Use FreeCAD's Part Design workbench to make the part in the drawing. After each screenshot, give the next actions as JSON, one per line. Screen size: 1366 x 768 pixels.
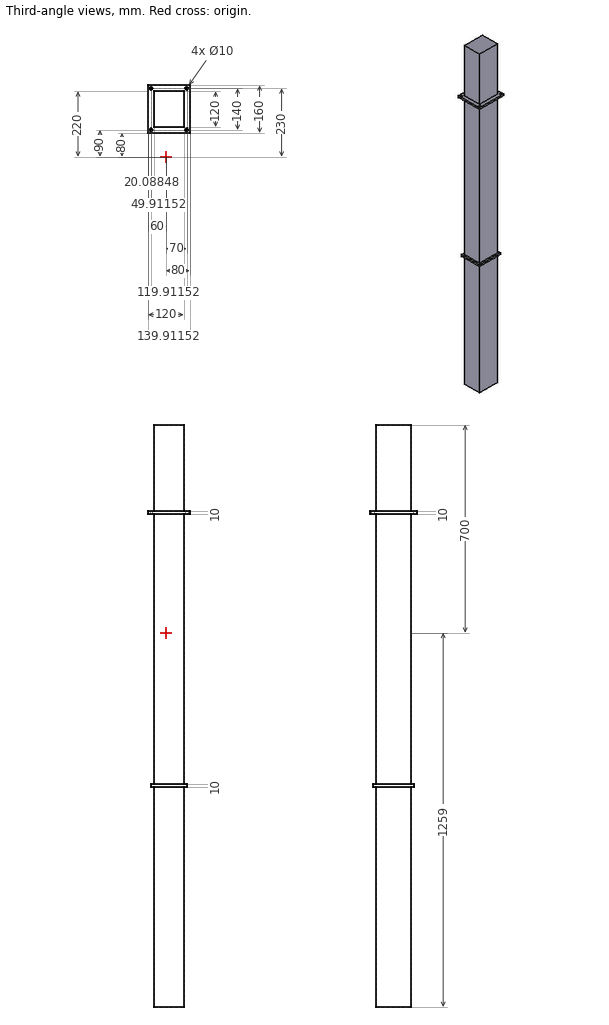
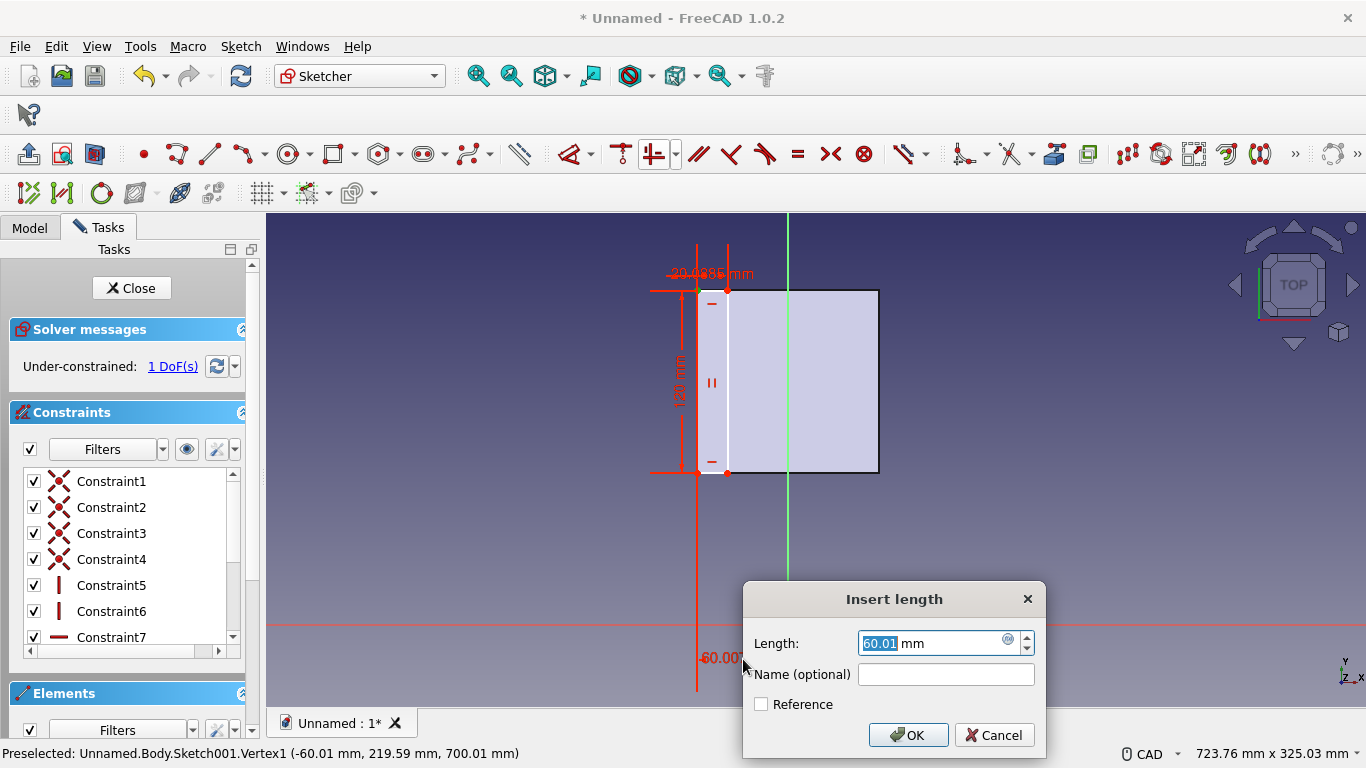
{"action": "type", "text": "60"}
{"action": "key", "text": "Return"}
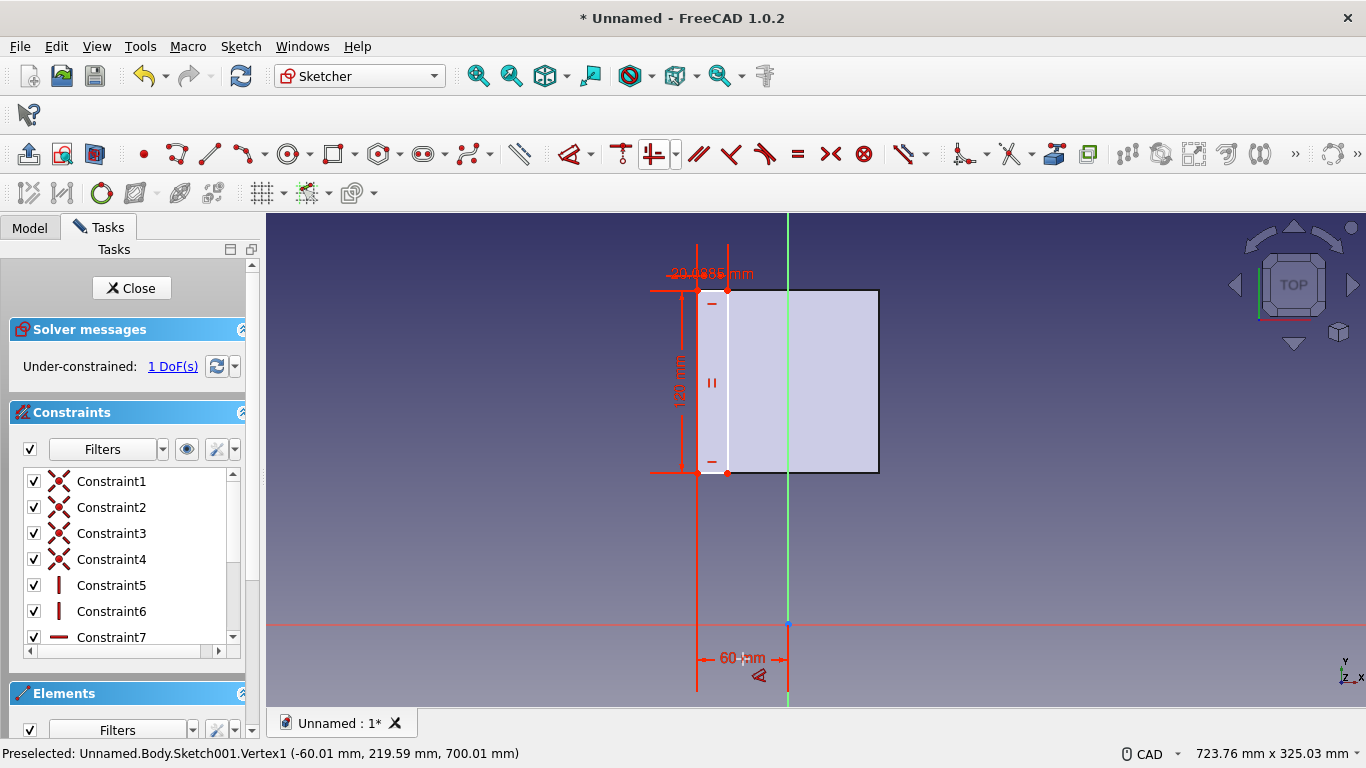
{"action": "left_click", "coordinate": [697, 291]}
{"action": "left_click", "coordinate": [822, 458]}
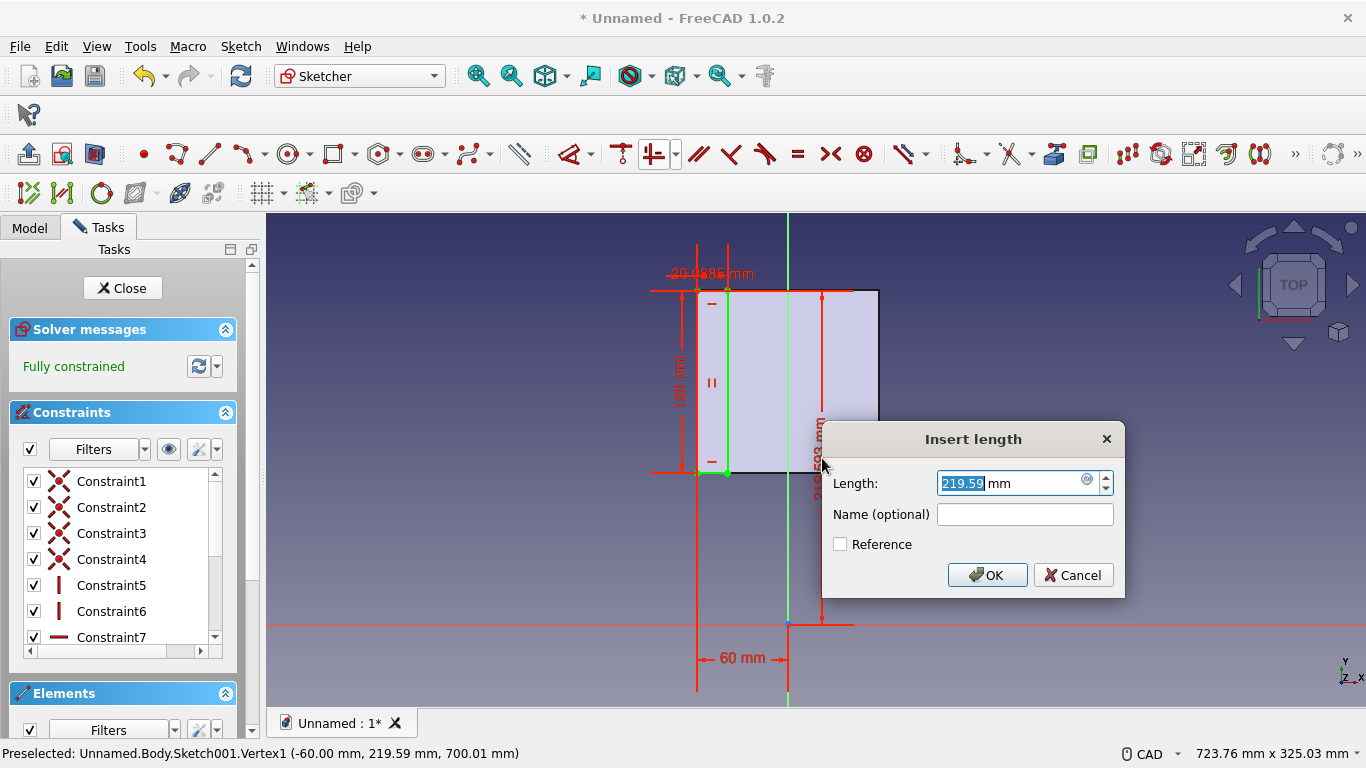
{"action": "type", "text": "220"}
{"action": "key", "text": "Return"}
{"action": "key", "text": "Escape"}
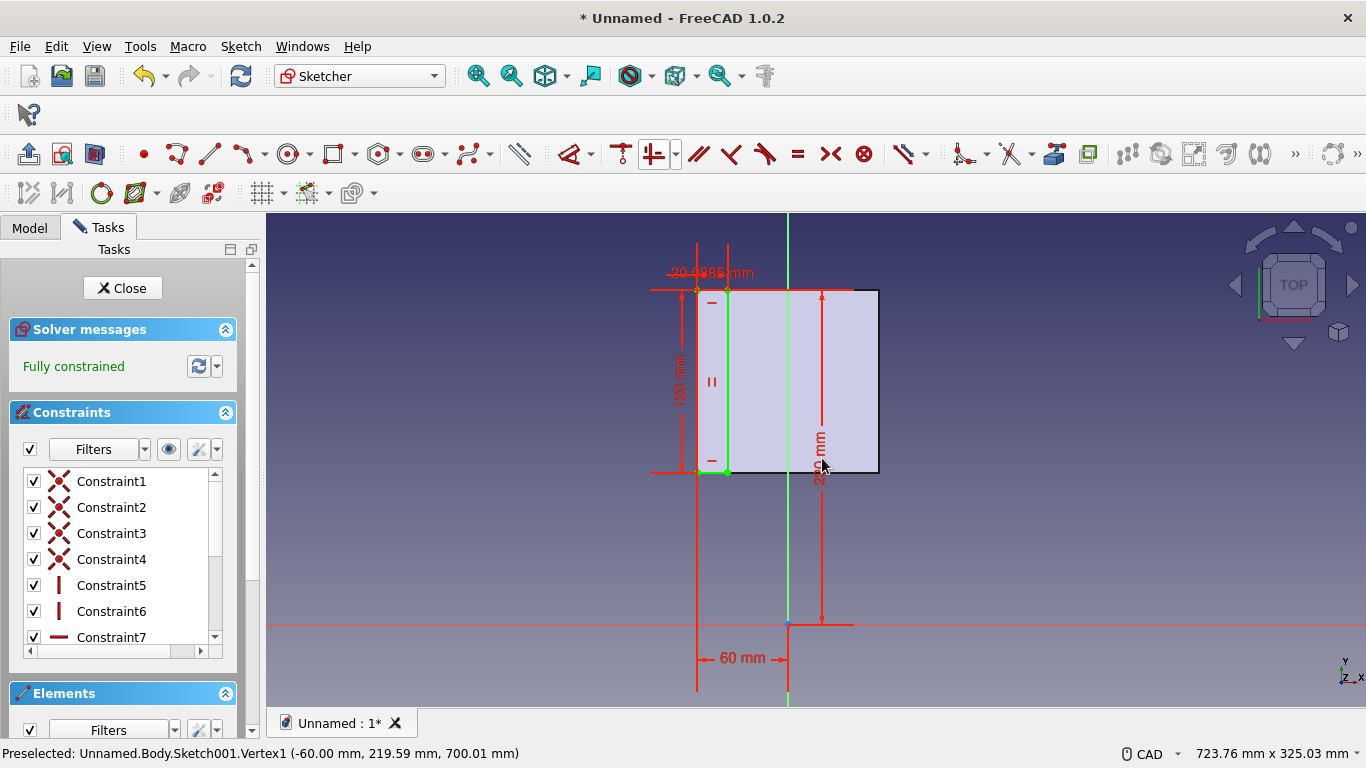
{"action": "left_click", "coordinate": [123, 288]}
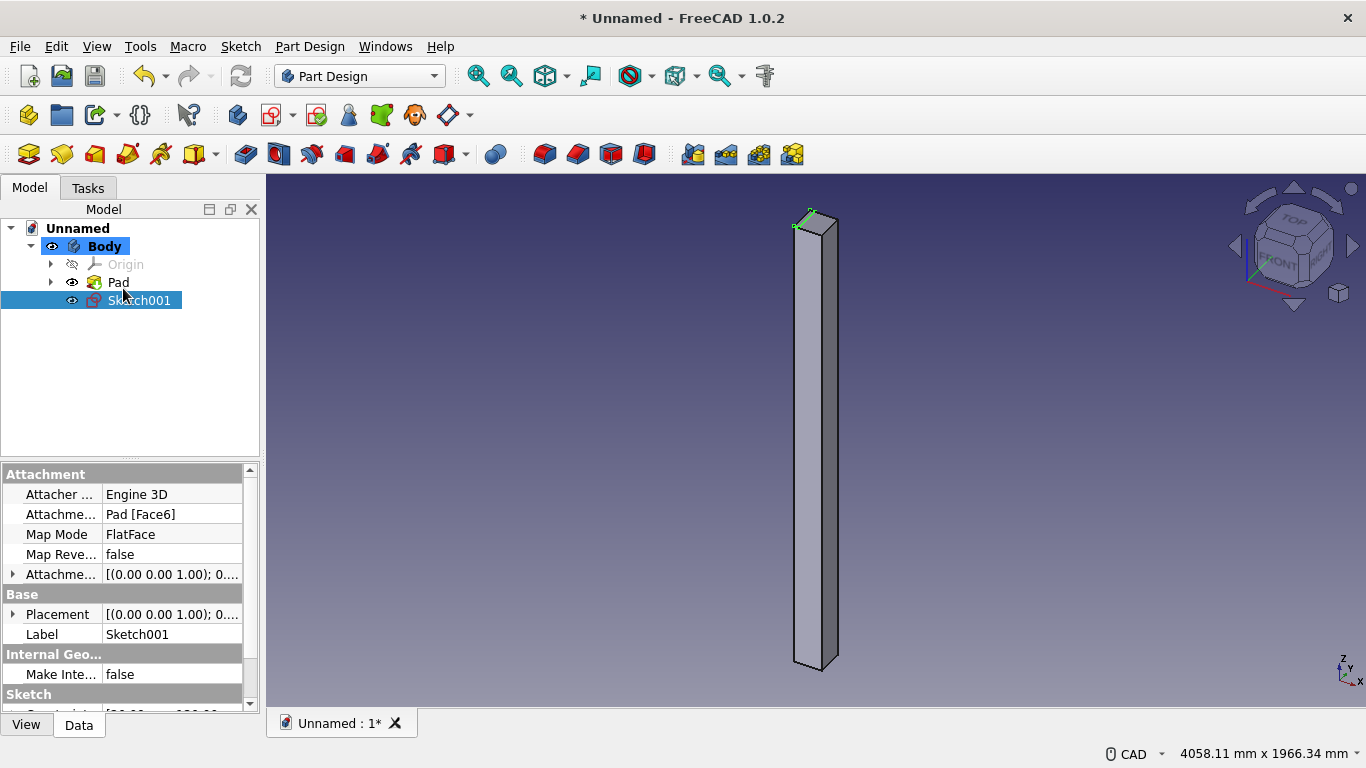
{"action": "left_click", "coordinate": [246, 154]}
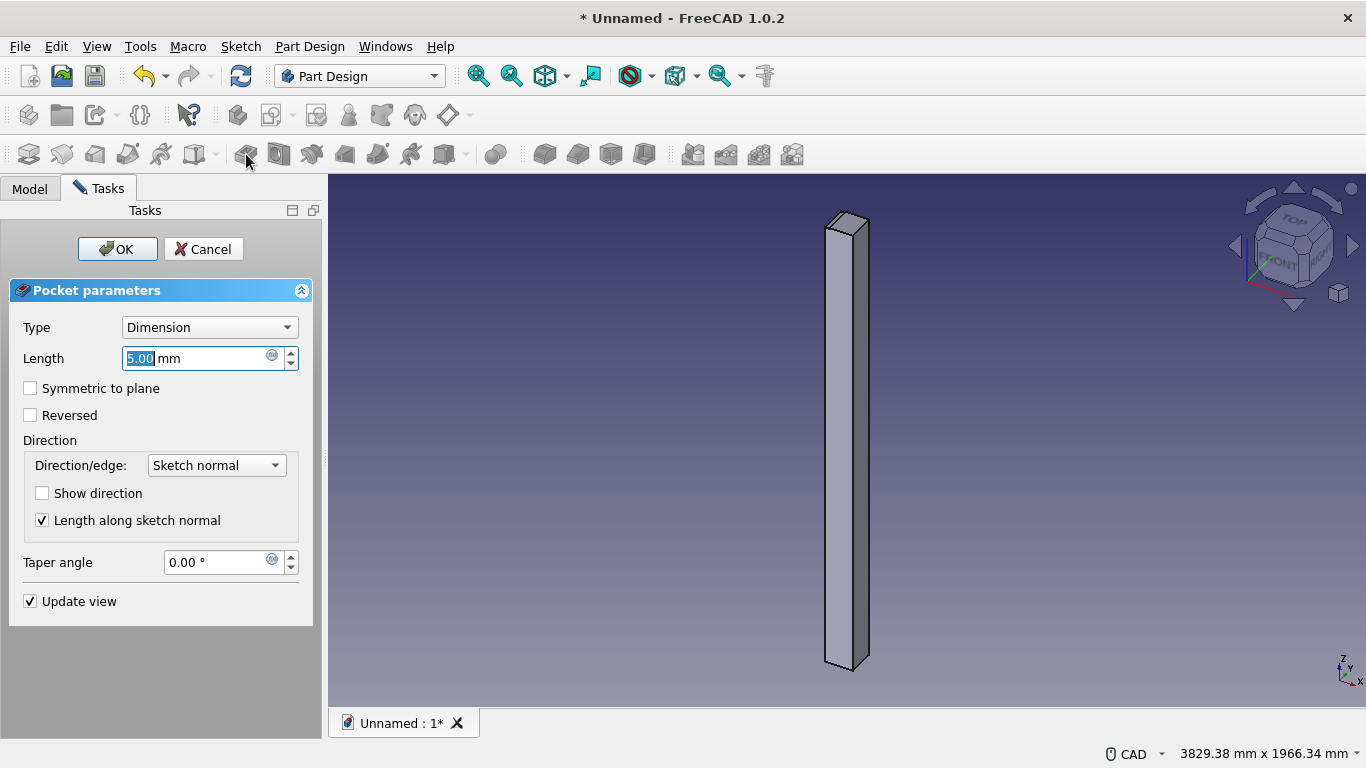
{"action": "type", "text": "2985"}
{"action": "key", "text": "Tab"}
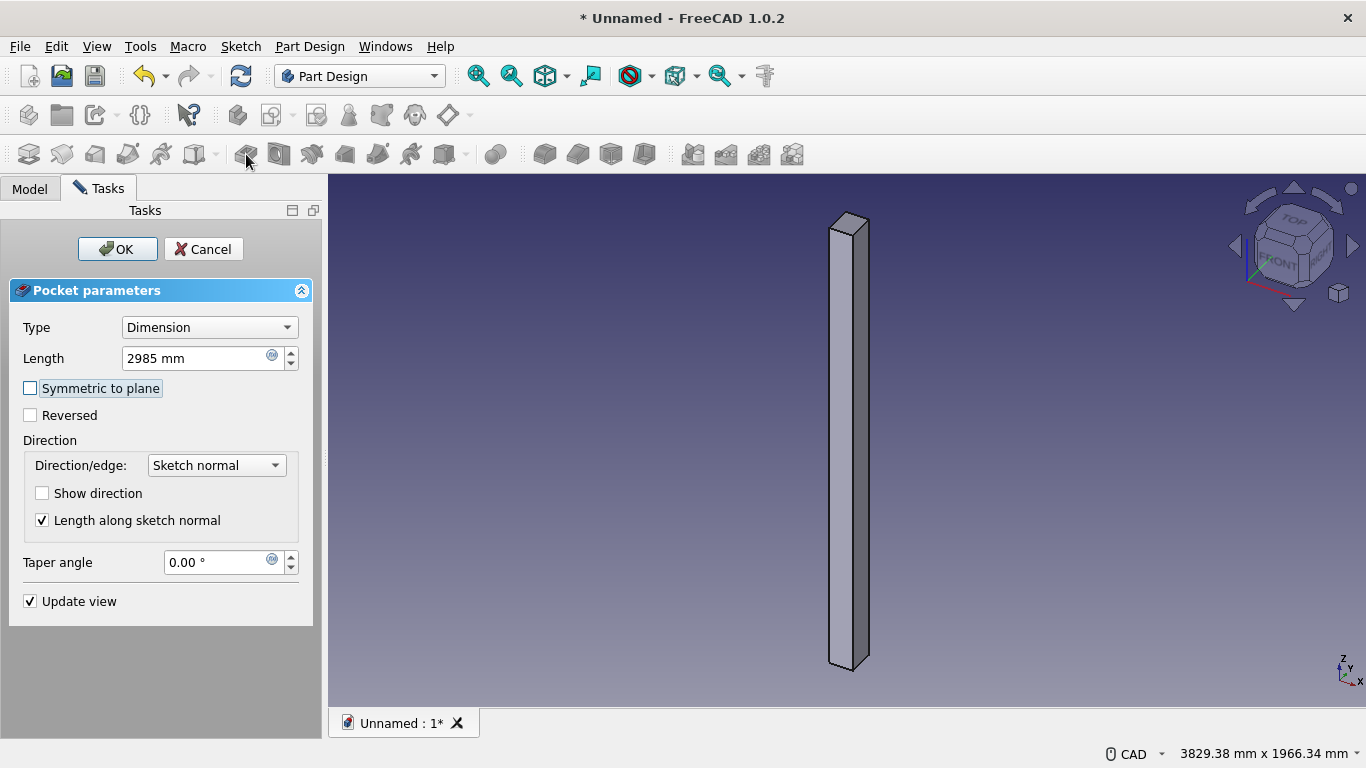
{"action": "left_click", "coordinate": [118, 249]}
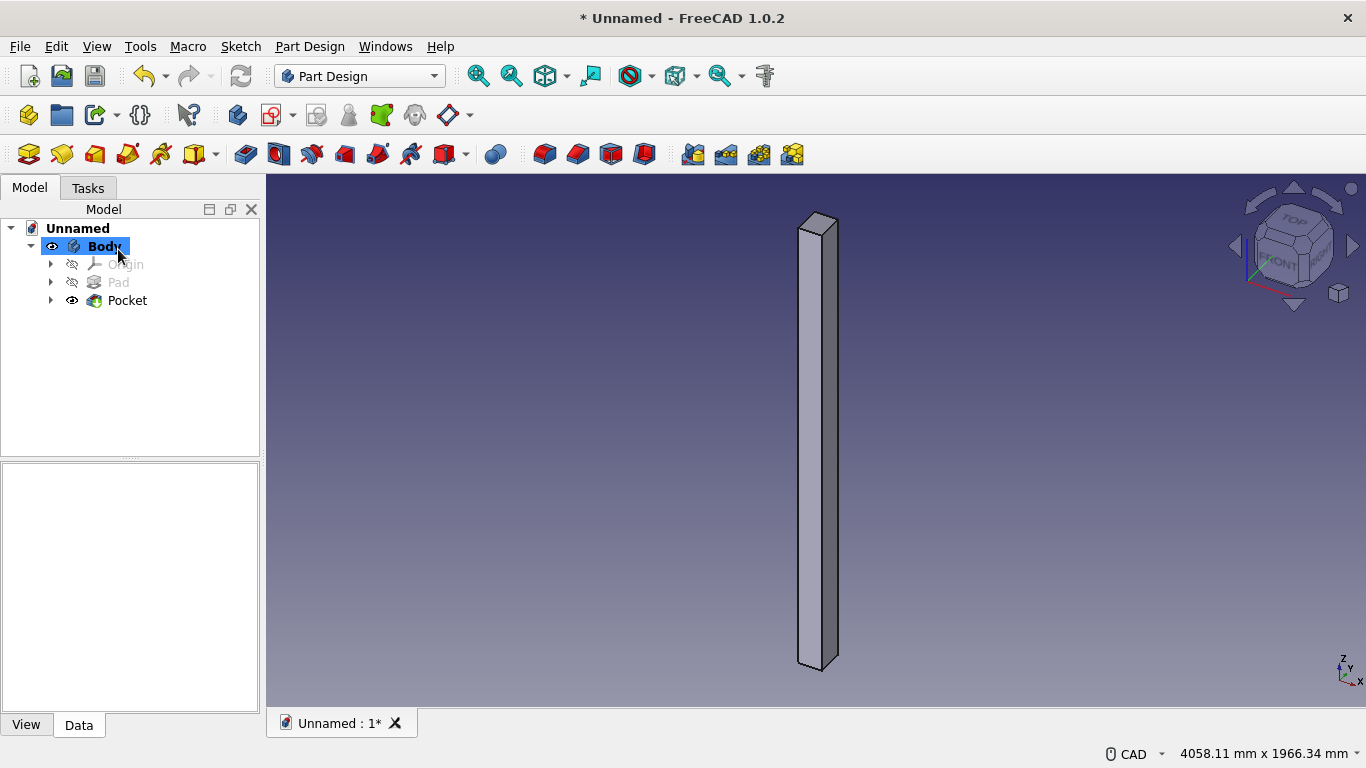
{"action": "left_click", "coordinate": [51, 264]}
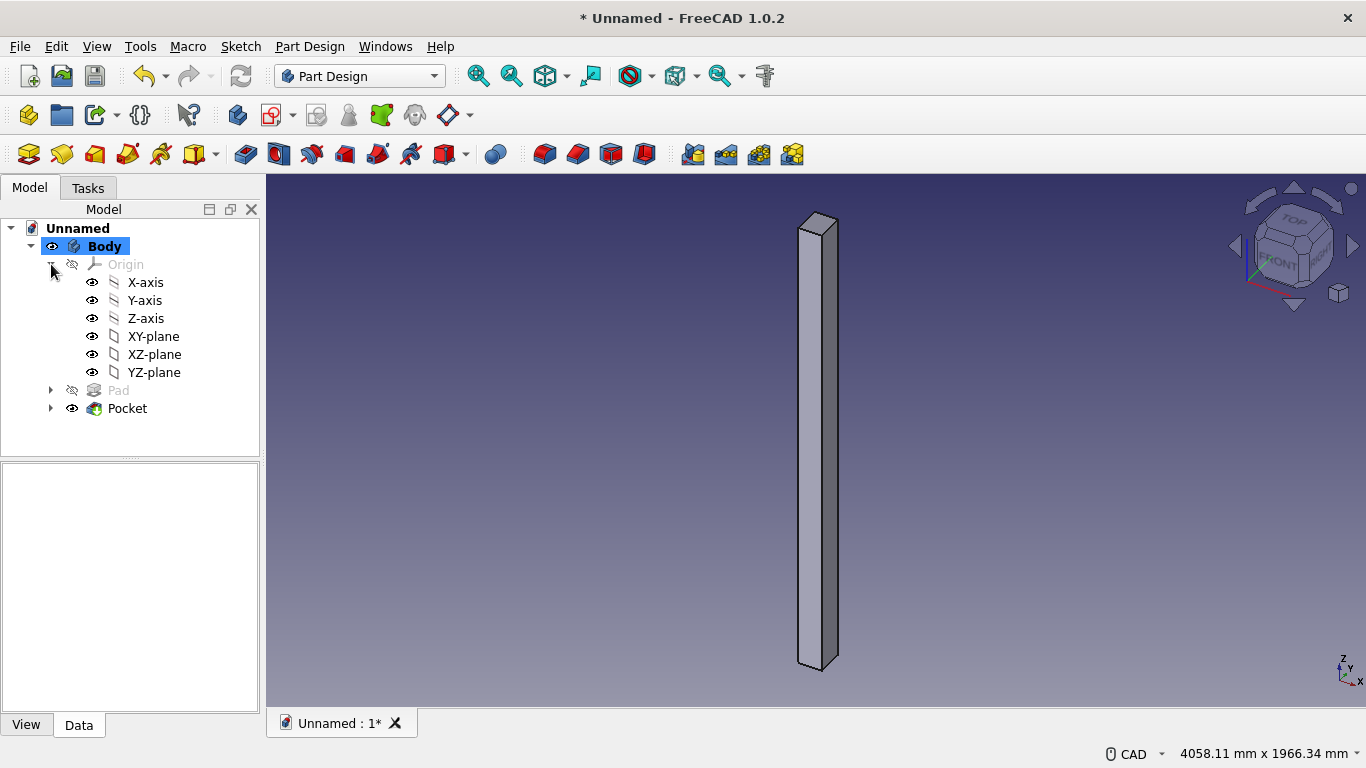
{"action": "left_click", "coordinate": [137, 336]}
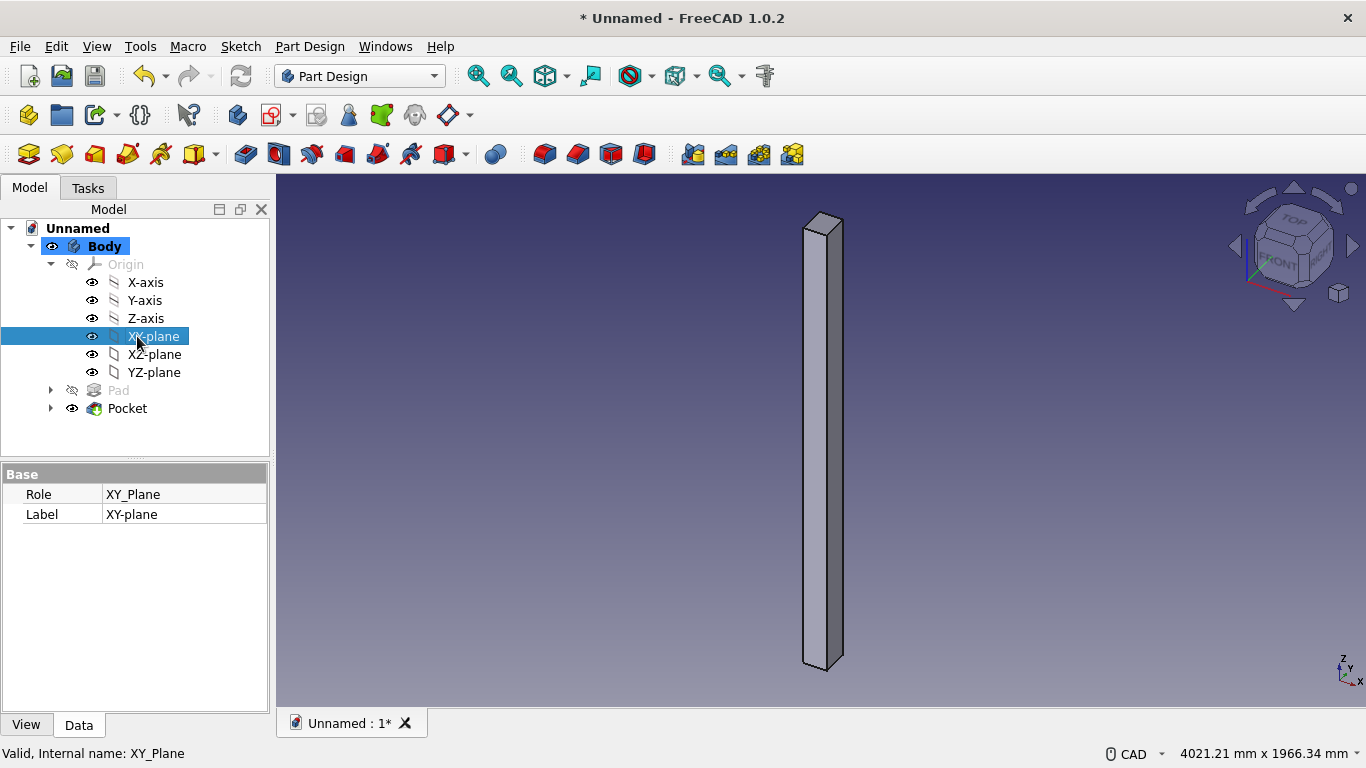
{"action": "left_click", "coordinate": [448, 116]}